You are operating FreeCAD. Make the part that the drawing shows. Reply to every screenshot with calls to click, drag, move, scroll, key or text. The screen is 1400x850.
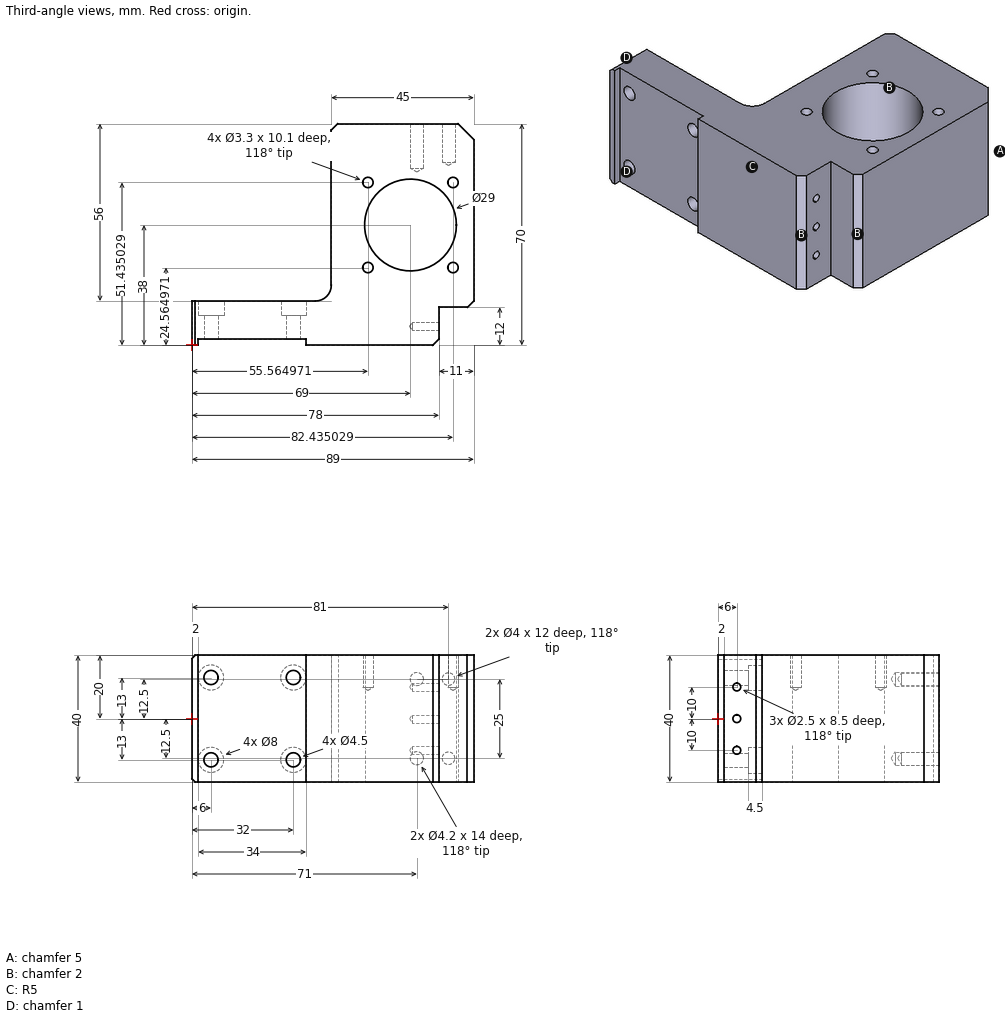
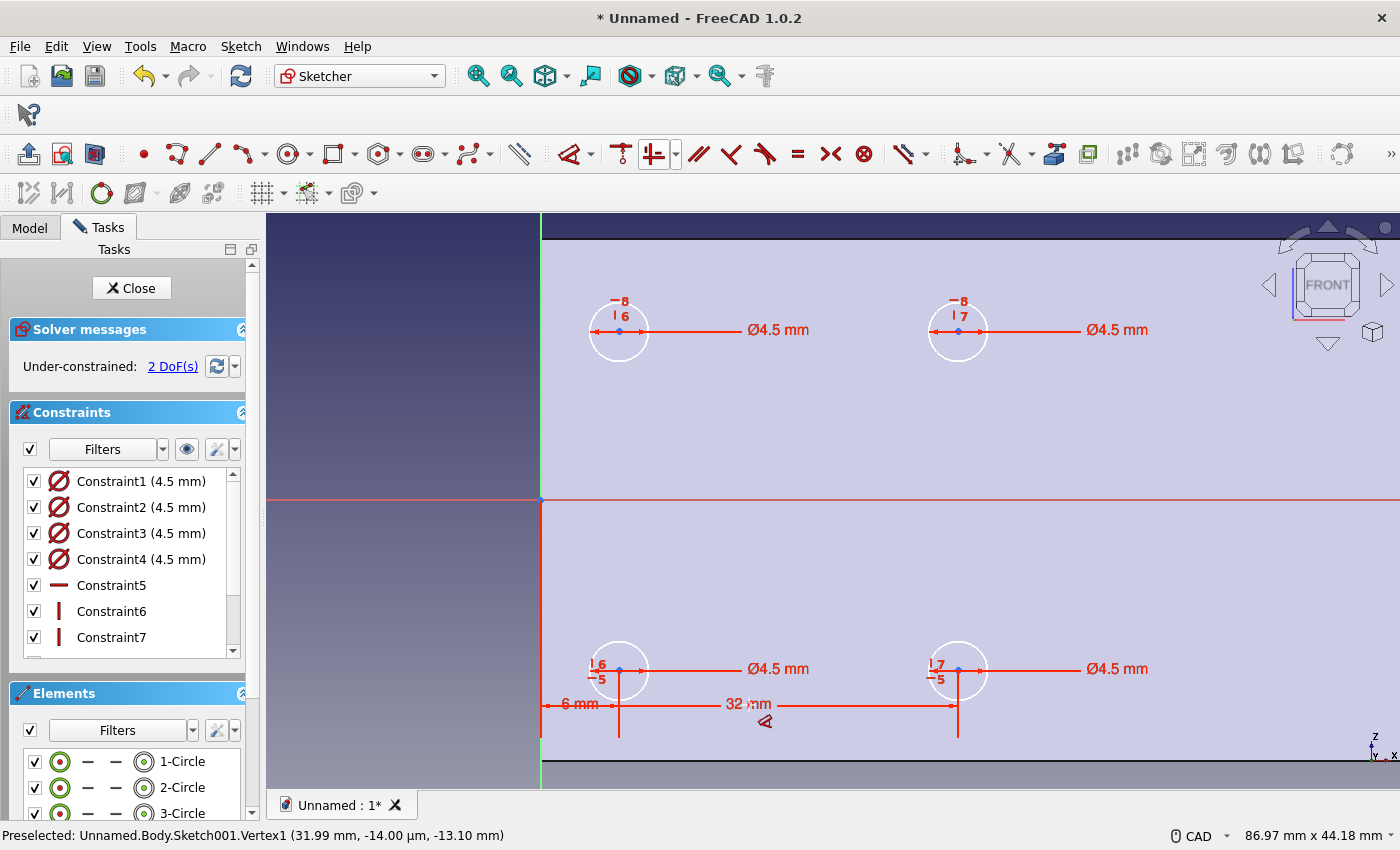
click(958, 671)
click(507, 586)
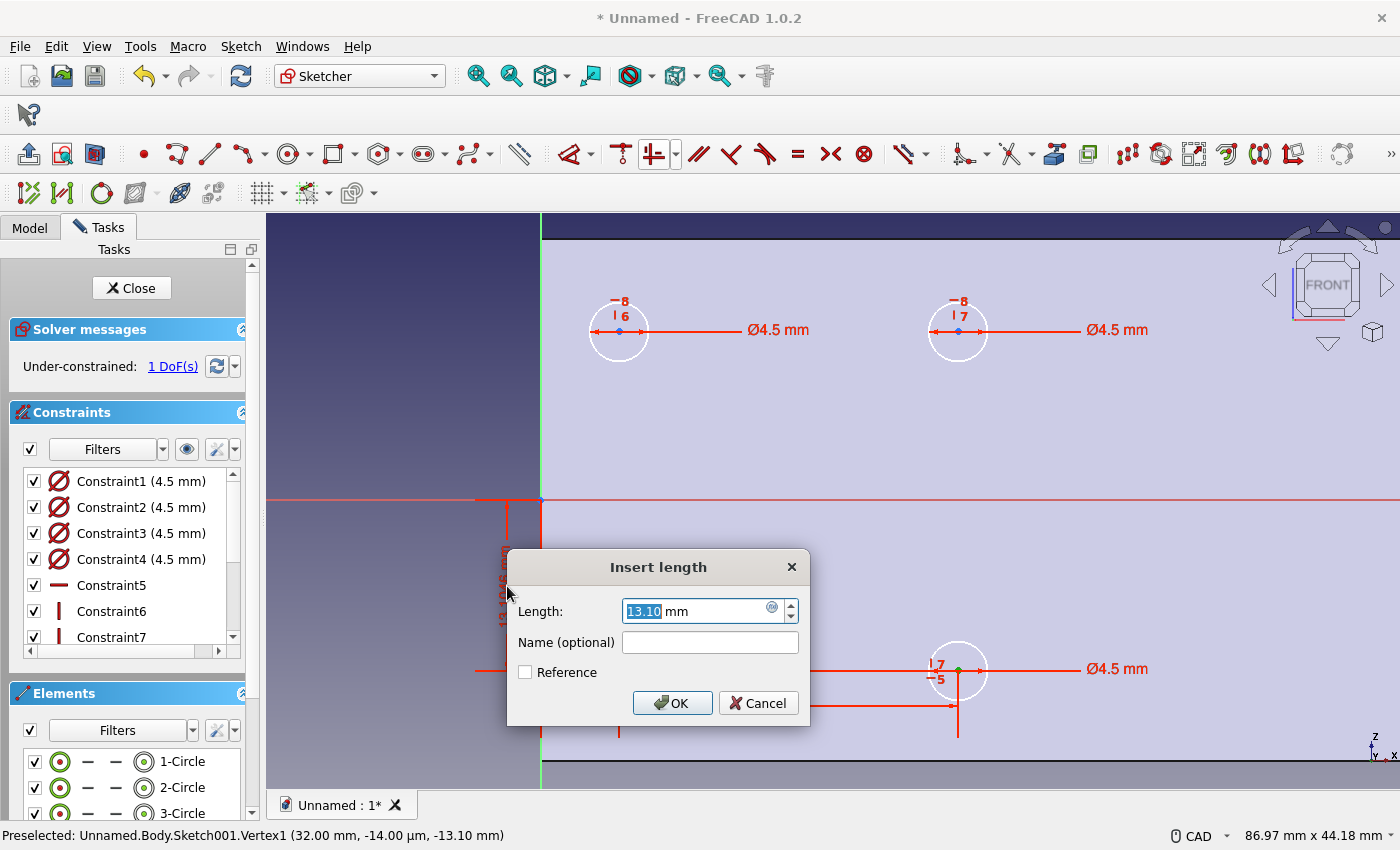
text(13)
key(Return)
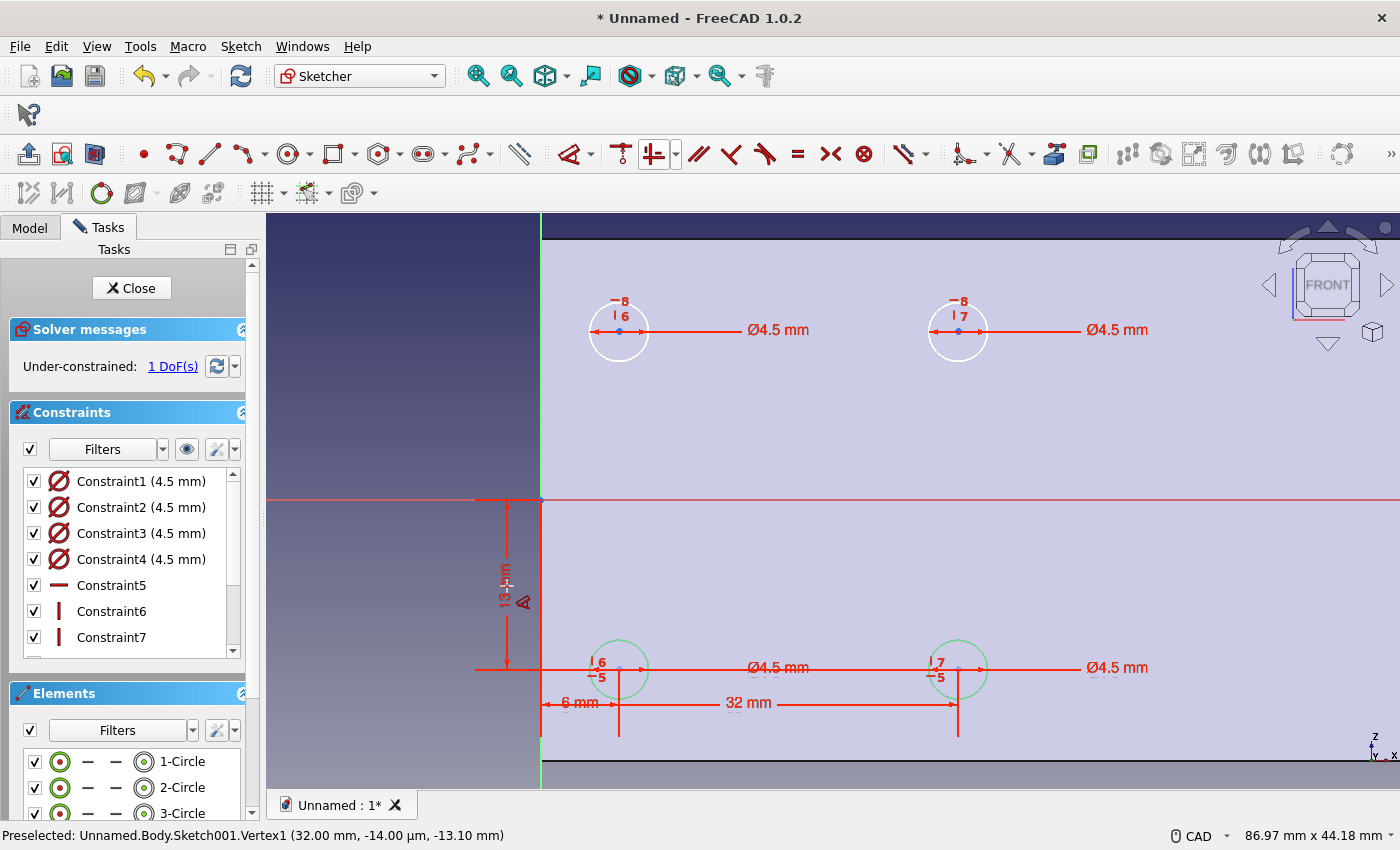
click(619, 332)
click(507, 416)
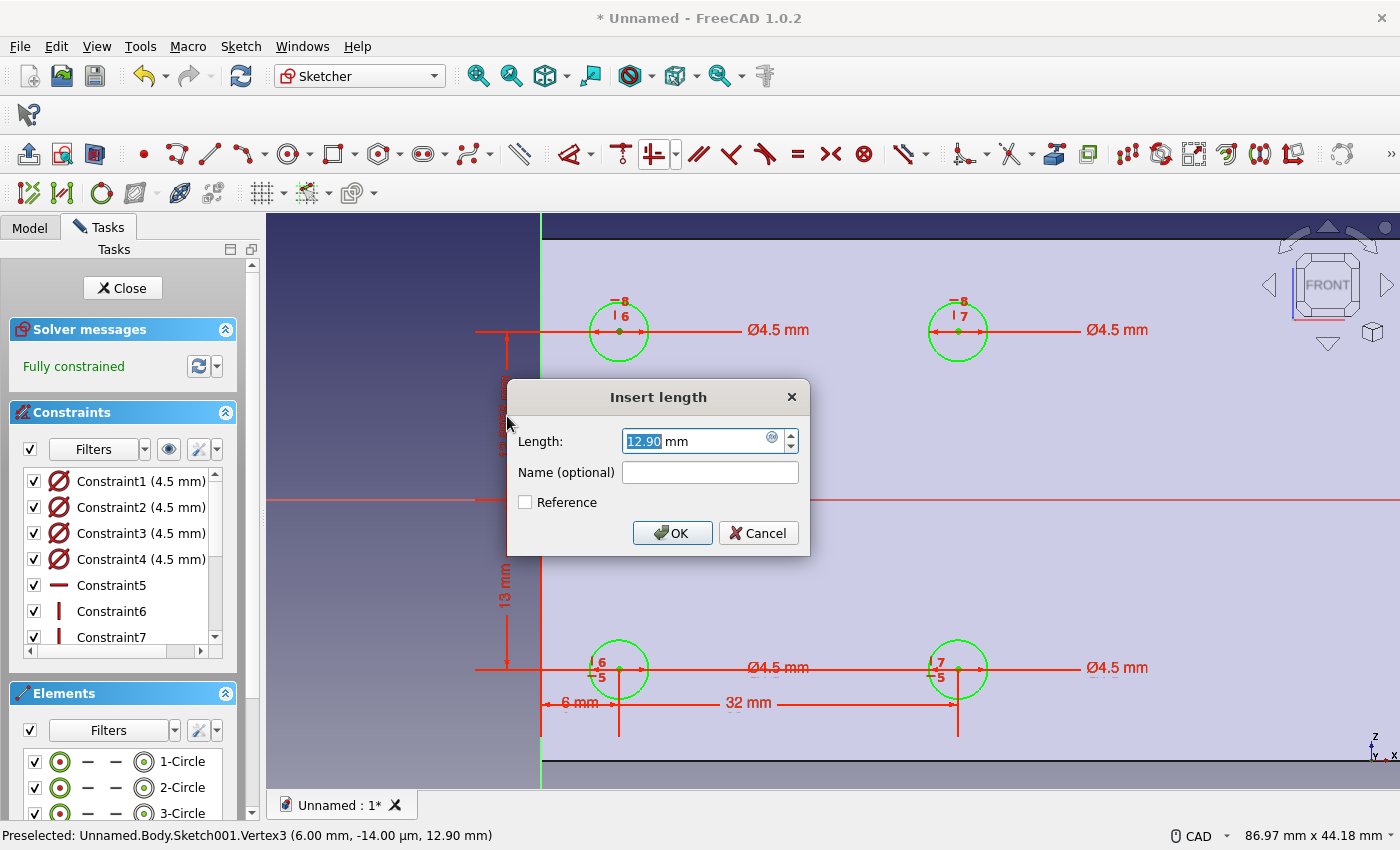
text(13)
key(Return)
key(Escape)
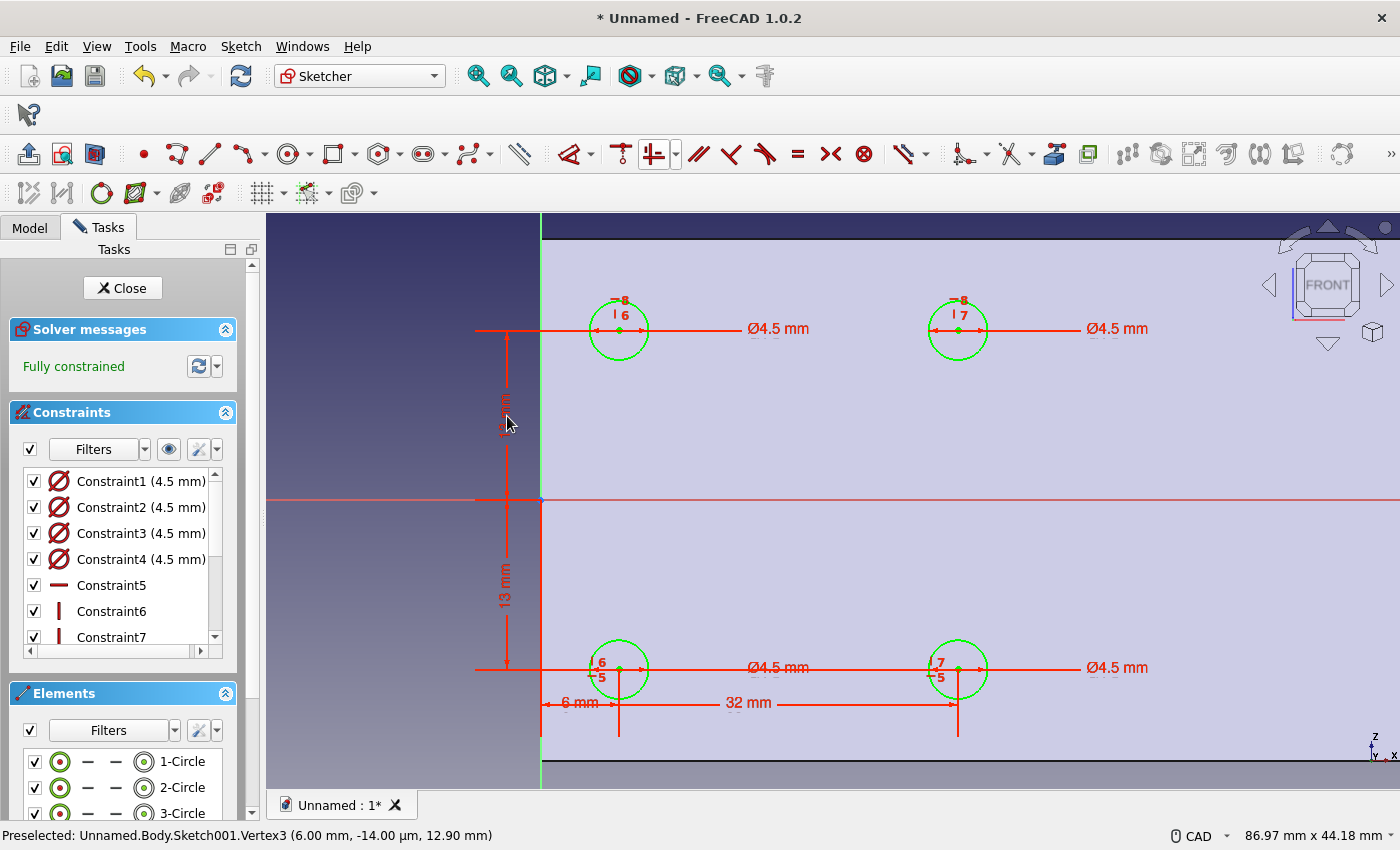
click(123, 288)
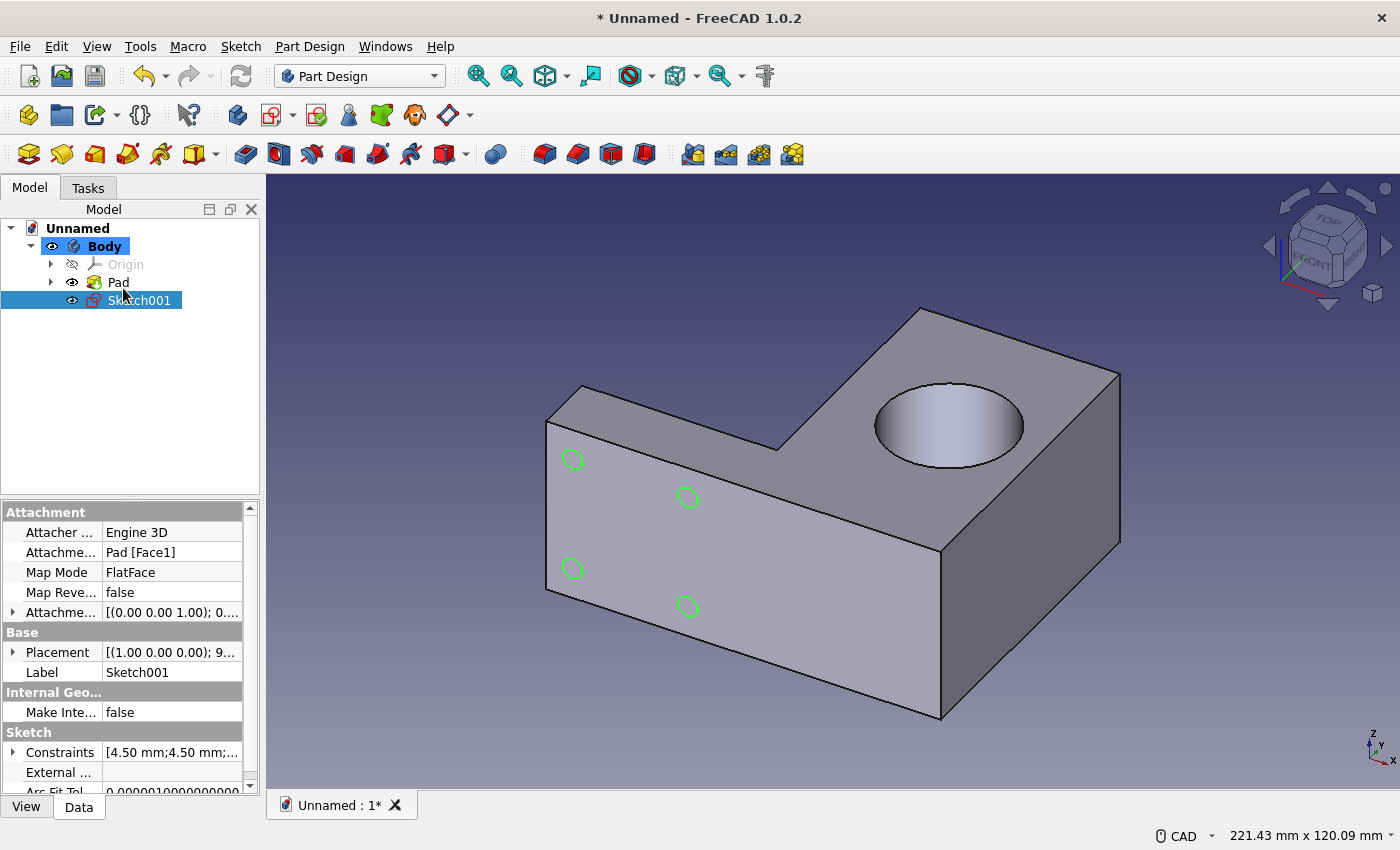
click(246, 154)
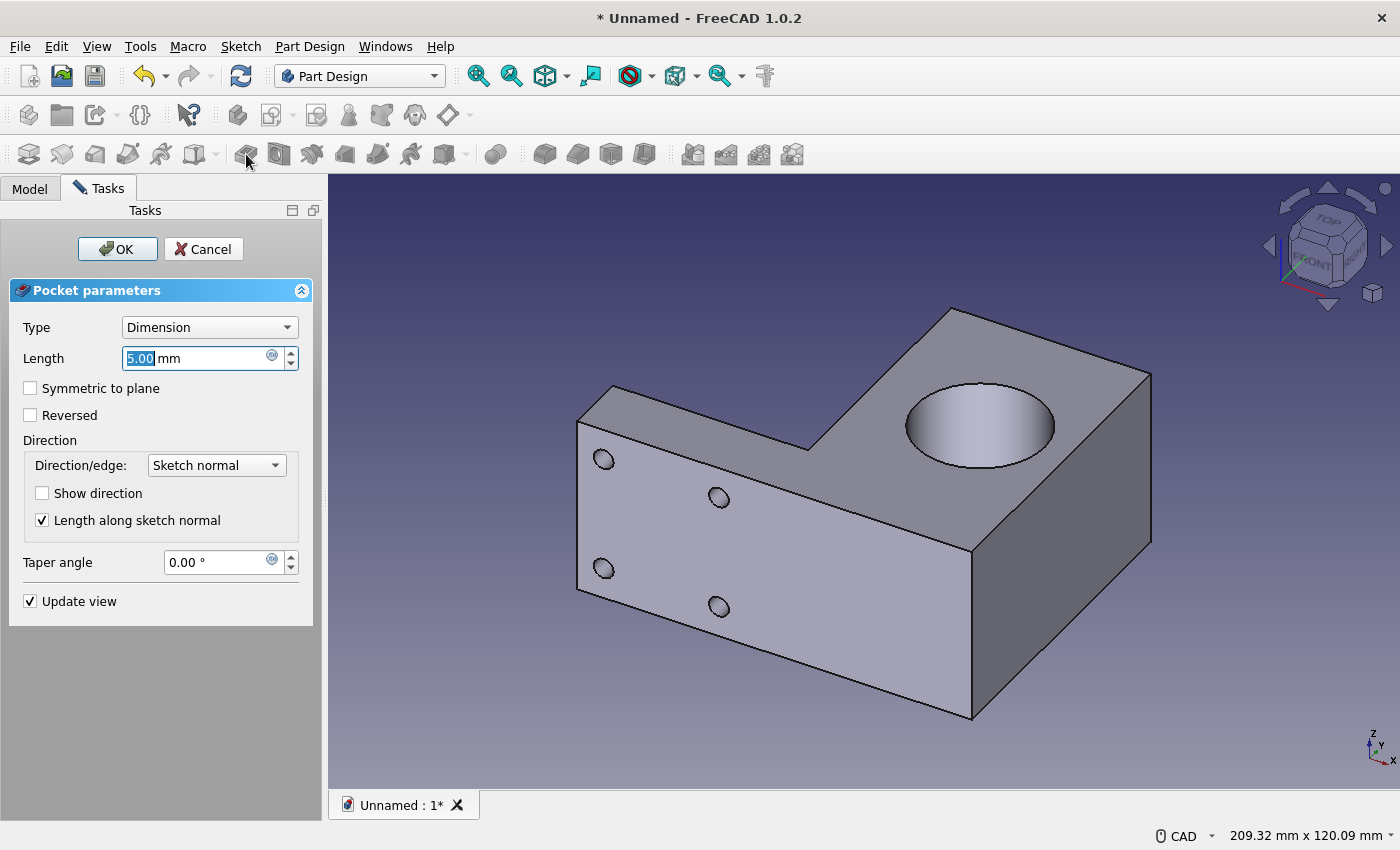
click(210, 328)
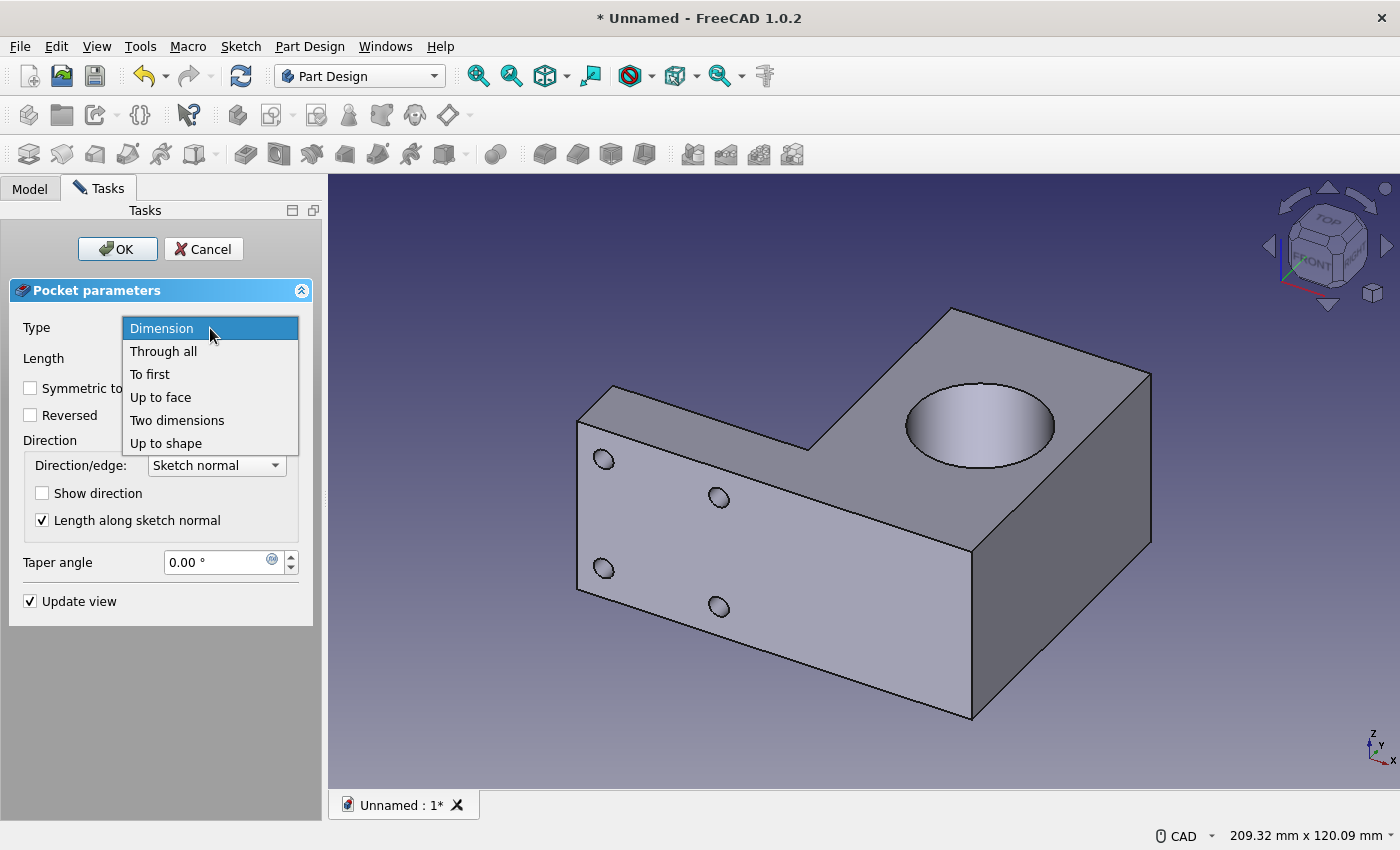
click(208, 352)